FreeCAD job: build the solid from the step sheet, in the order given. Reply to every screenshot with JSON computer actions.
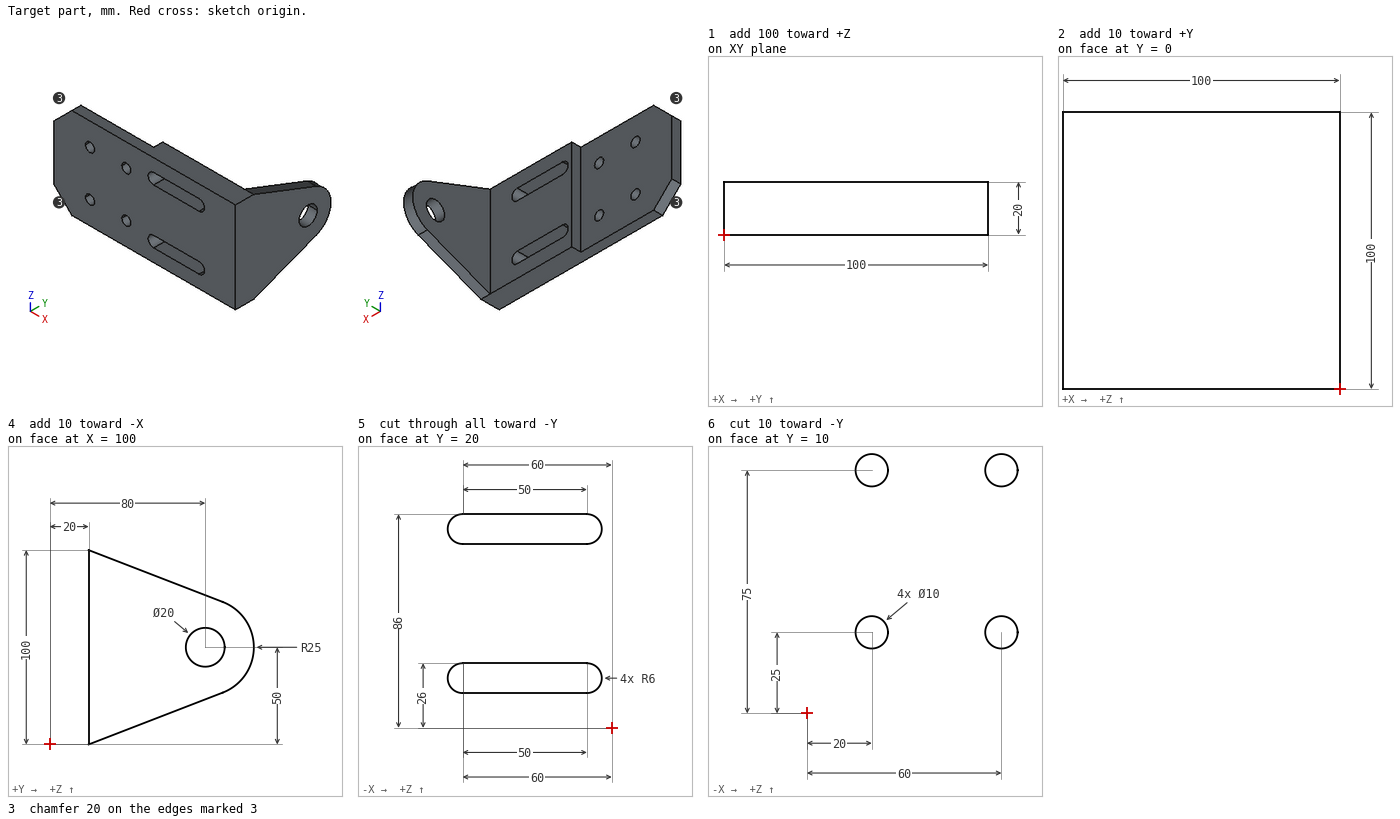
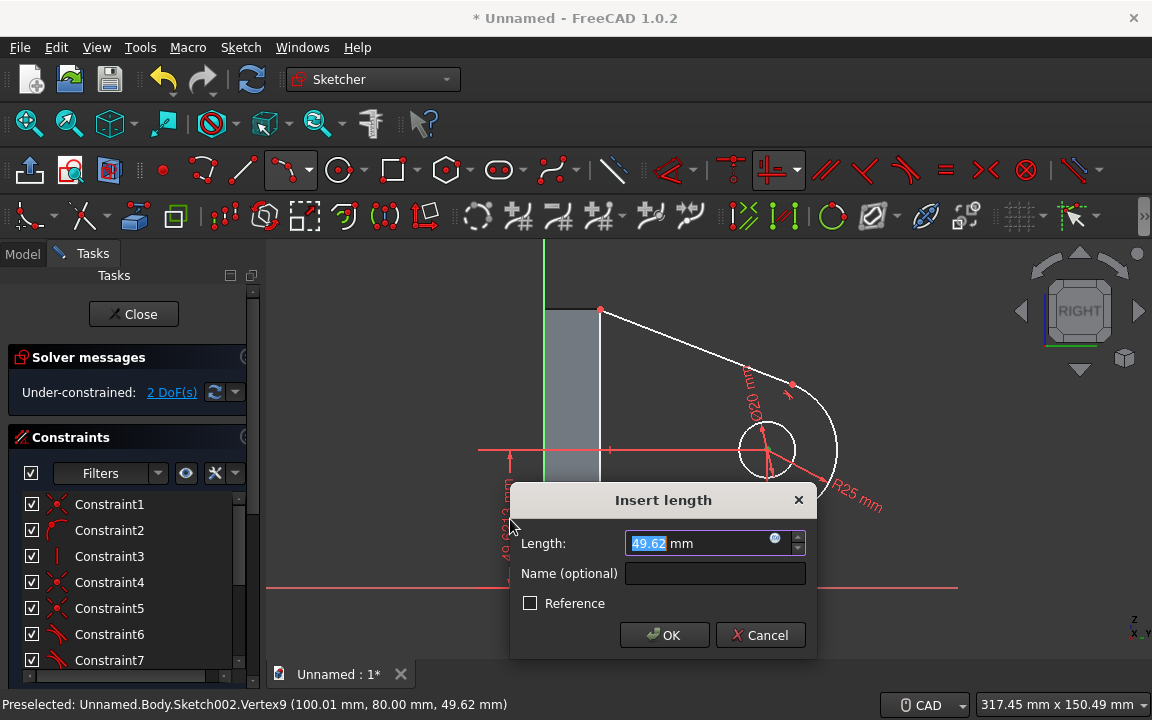
{"action": "type", "text": "50"}
{"action": "key", "text": "Return"}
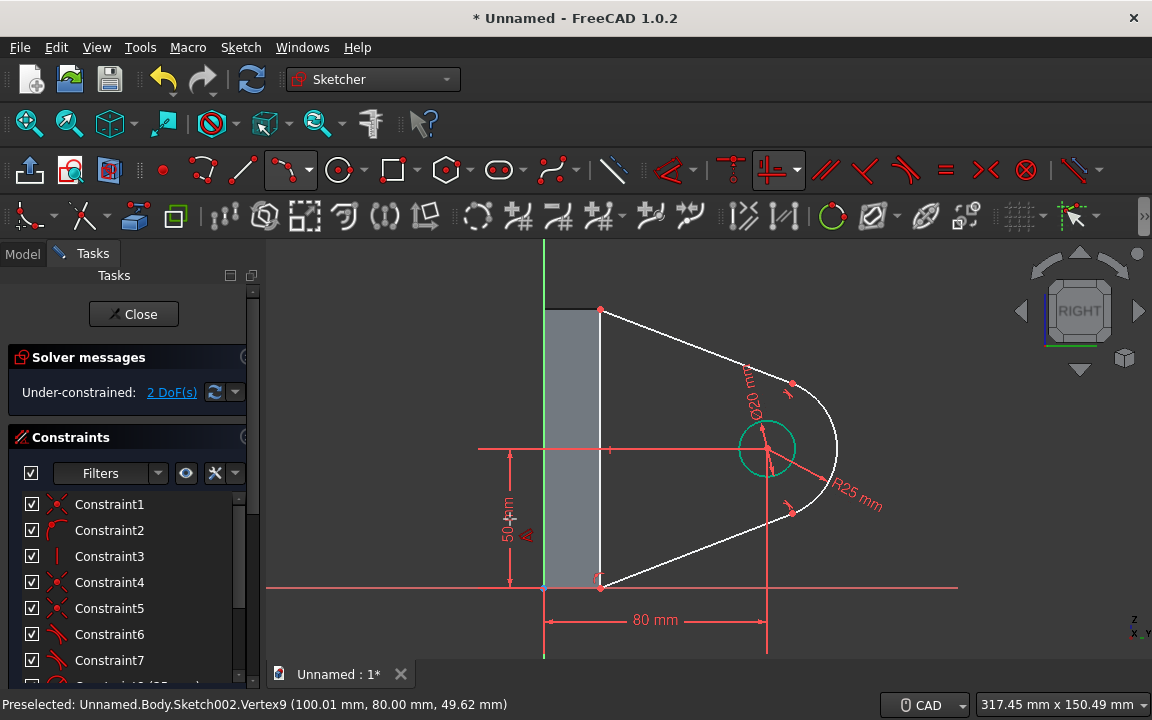
{"action": "left_click", "coordinate": [600, 393]}
{"action": "left_click", "coordinate": [566, 449]}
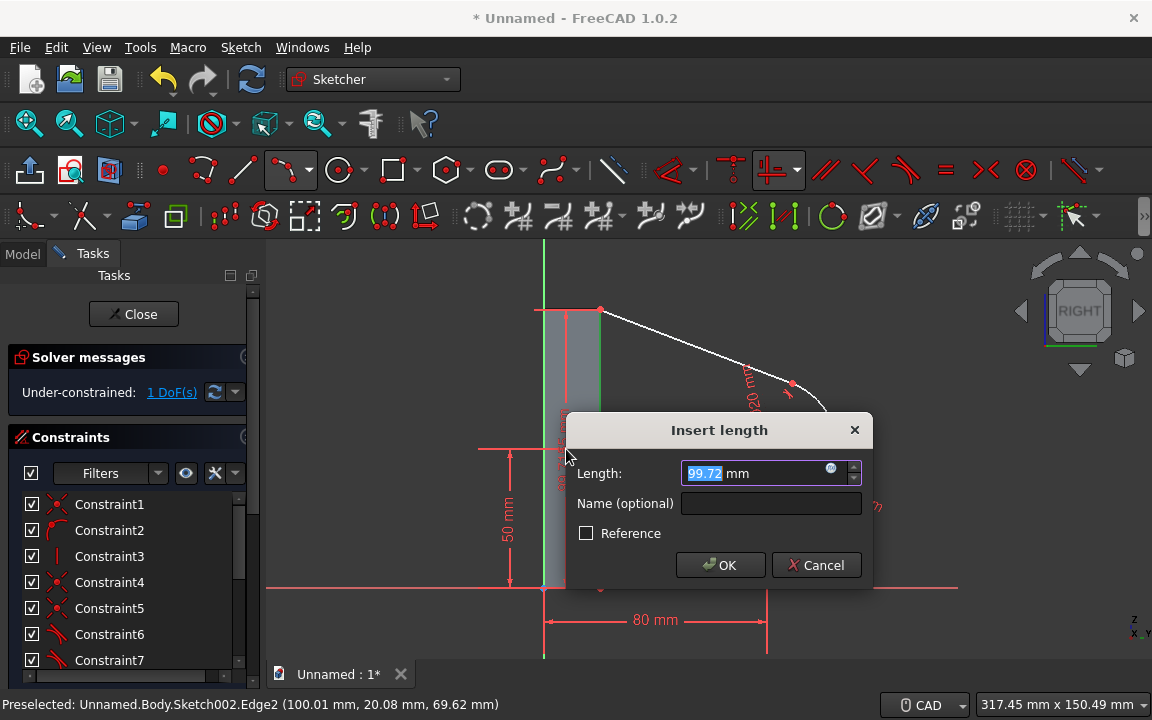
{"action": "type", "text": "100"}
{"action": "key", "text": "Return"}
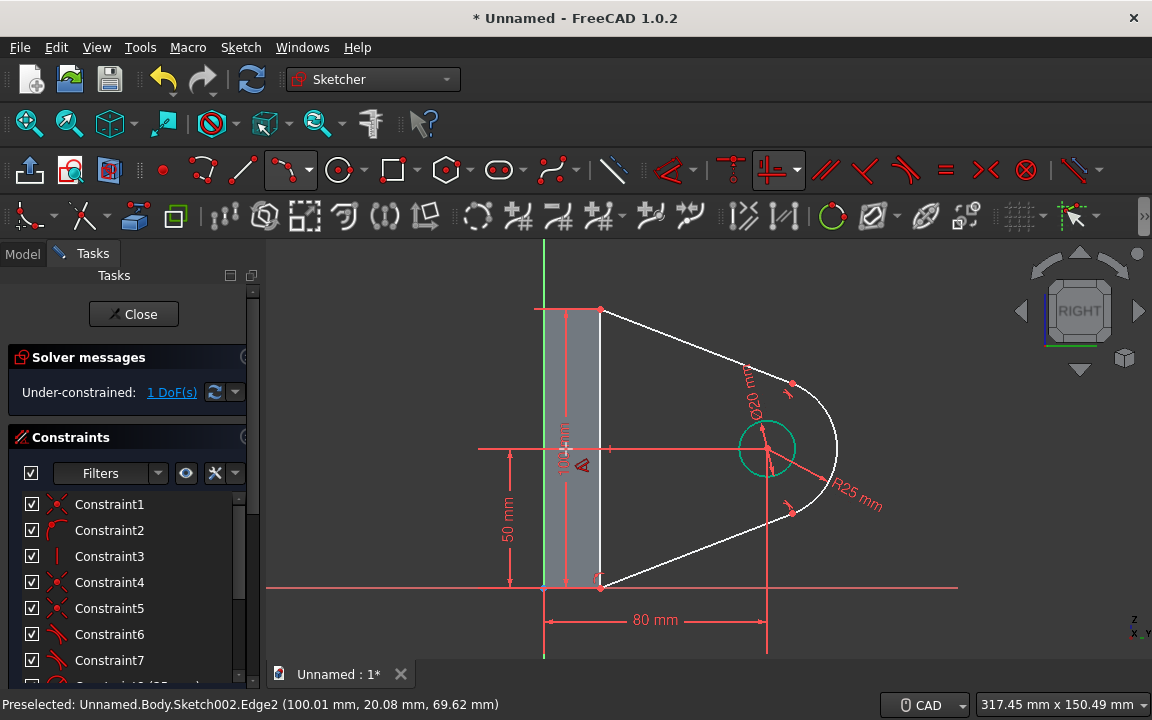
{"action": "left_click", "coordinate": [600, 309]}
{"action": "left_click", "coordinate": [572, 622]}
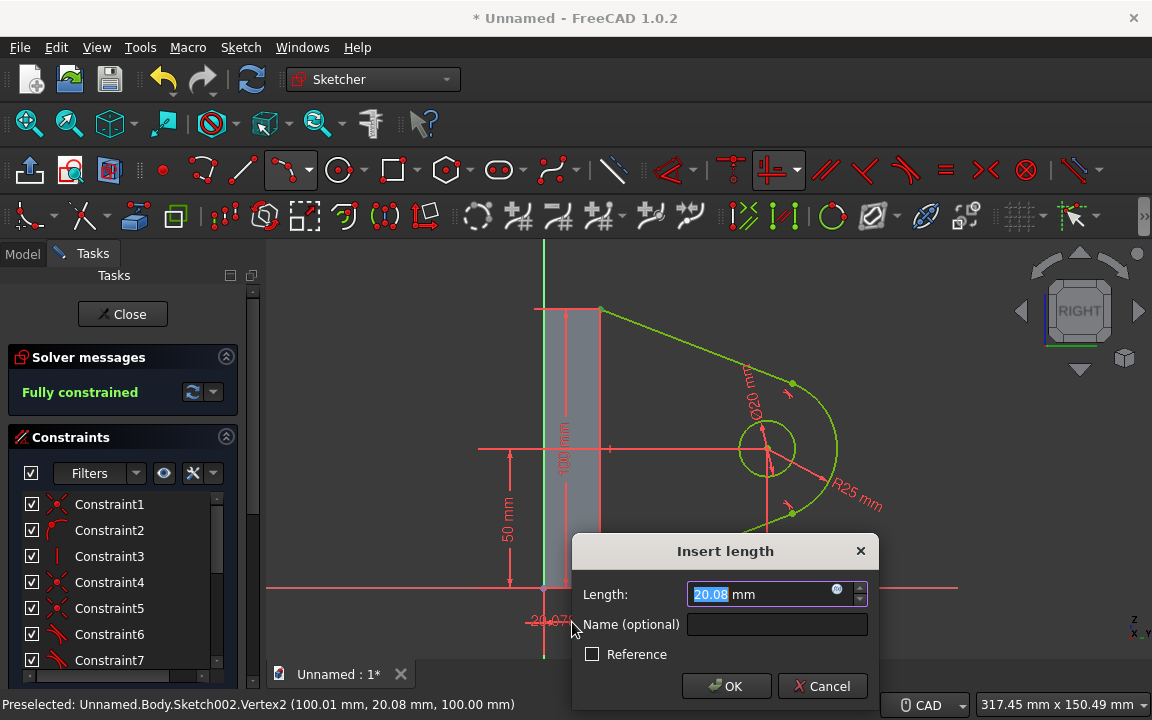
{"action": "type", "text": "20"}
{"action": "key", "text": "Return"}
{"action": "key", "text": "Escape"}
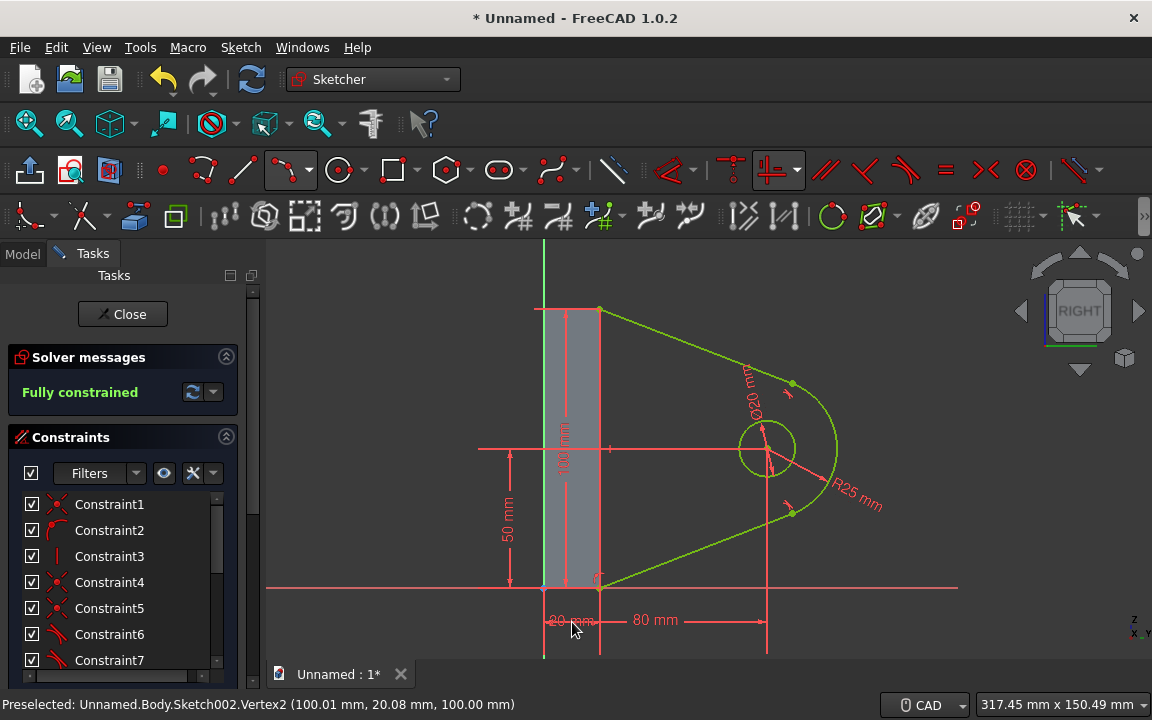
{"action": "left_click", "coordinate": [123, 314]}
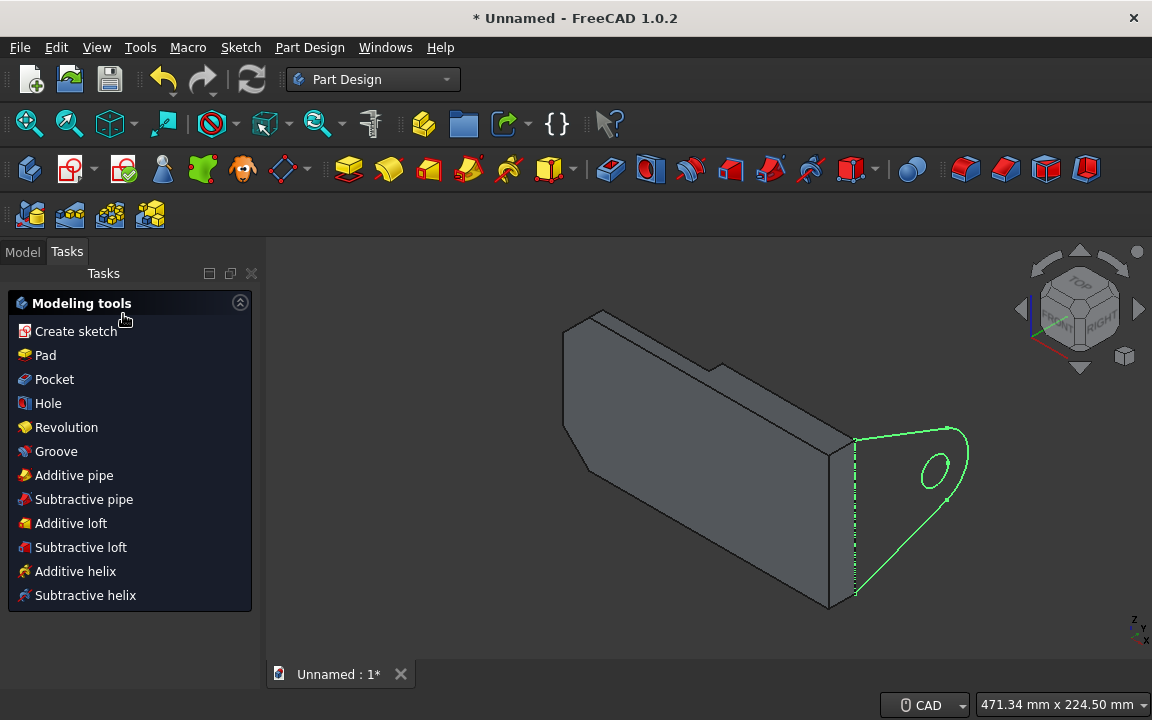
{"action": "left_click", "coordinate": [350, 170]}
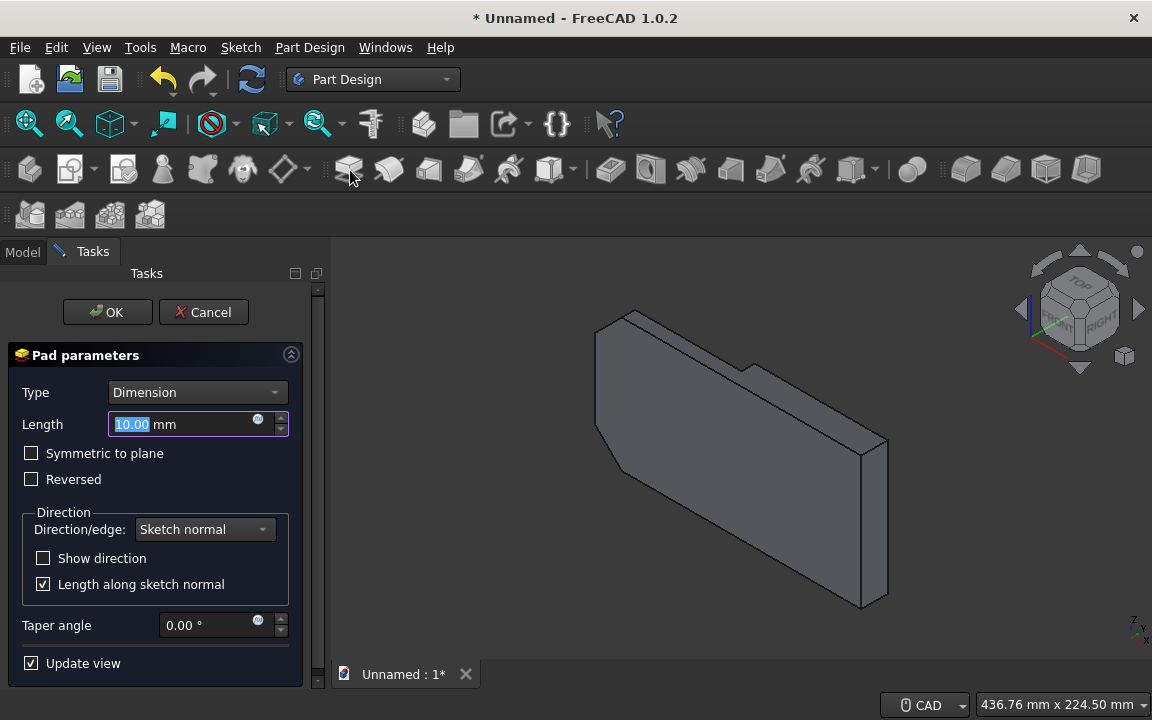
{"action": "type", "text": "10"}
{"action": "key", "text": "Tab"}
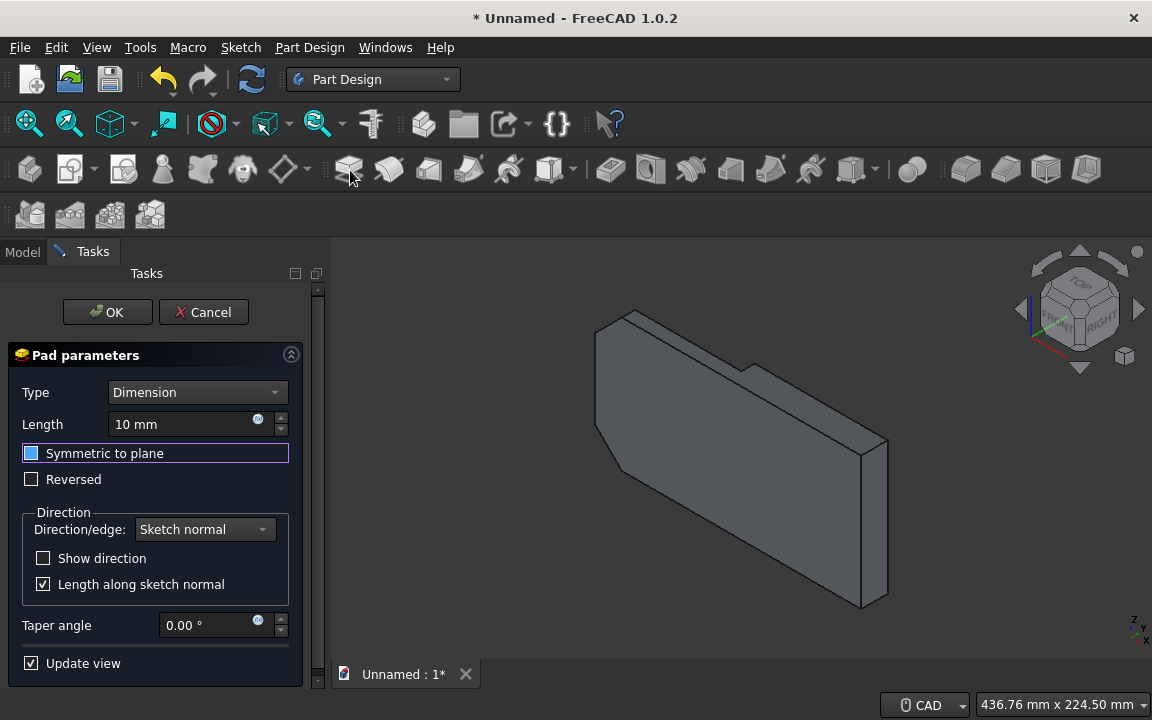
{"action": "left_click", "coordinate": [30, 479]}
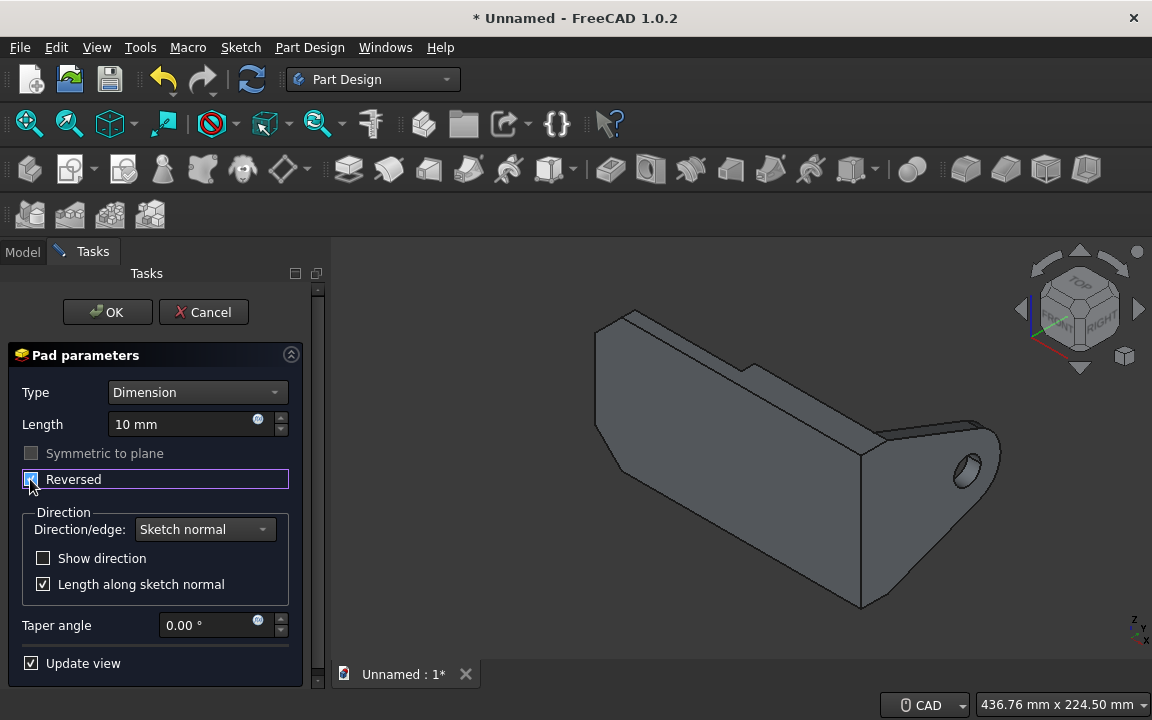
{"action": "left_click", "coordinate": [108, 312]}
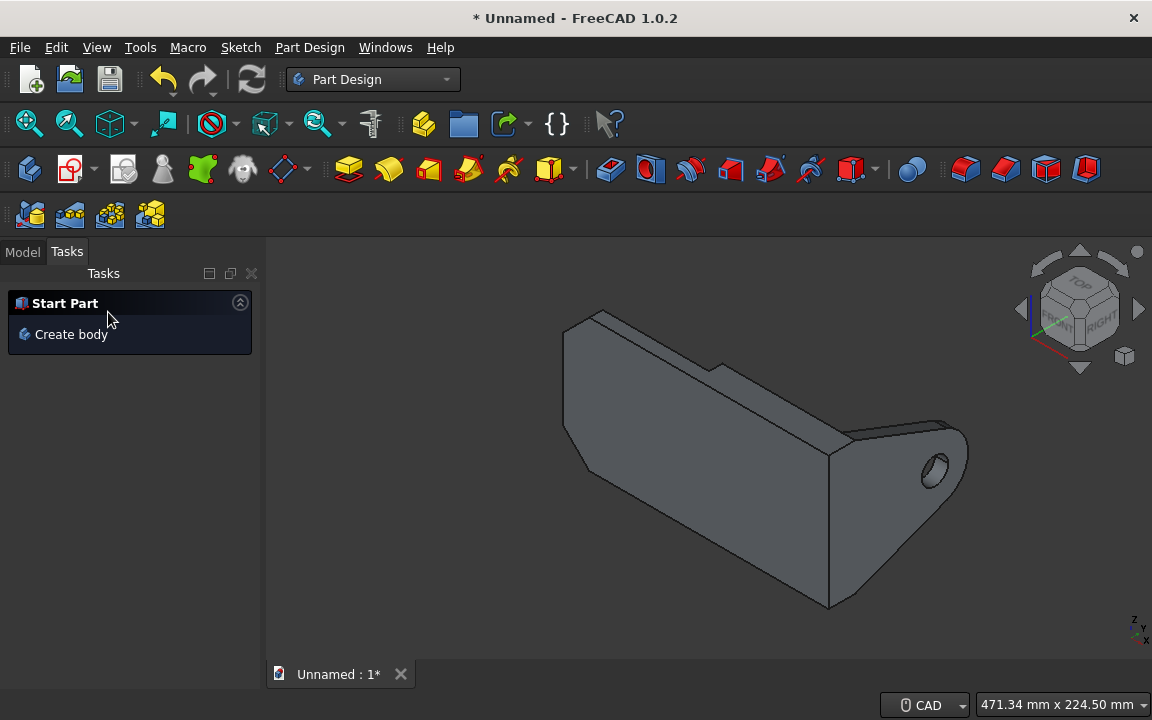
{"action": "left_click", "coordinate": [30, 124]}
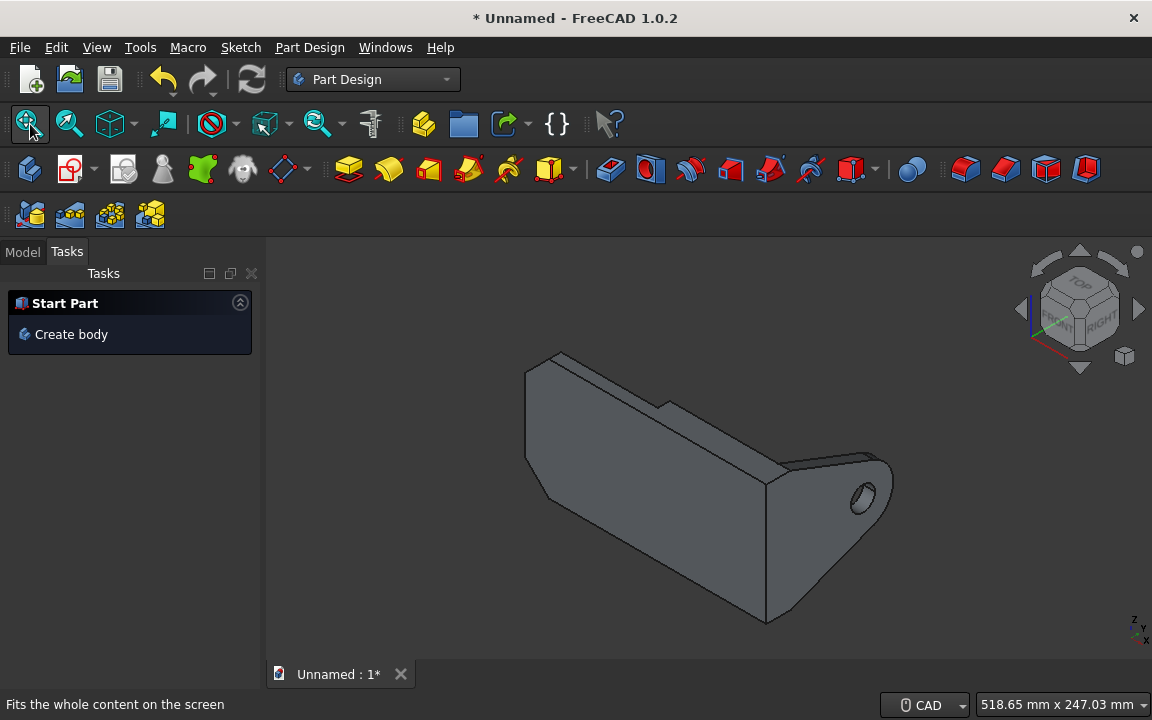
{"action": "key", "text": "4"}